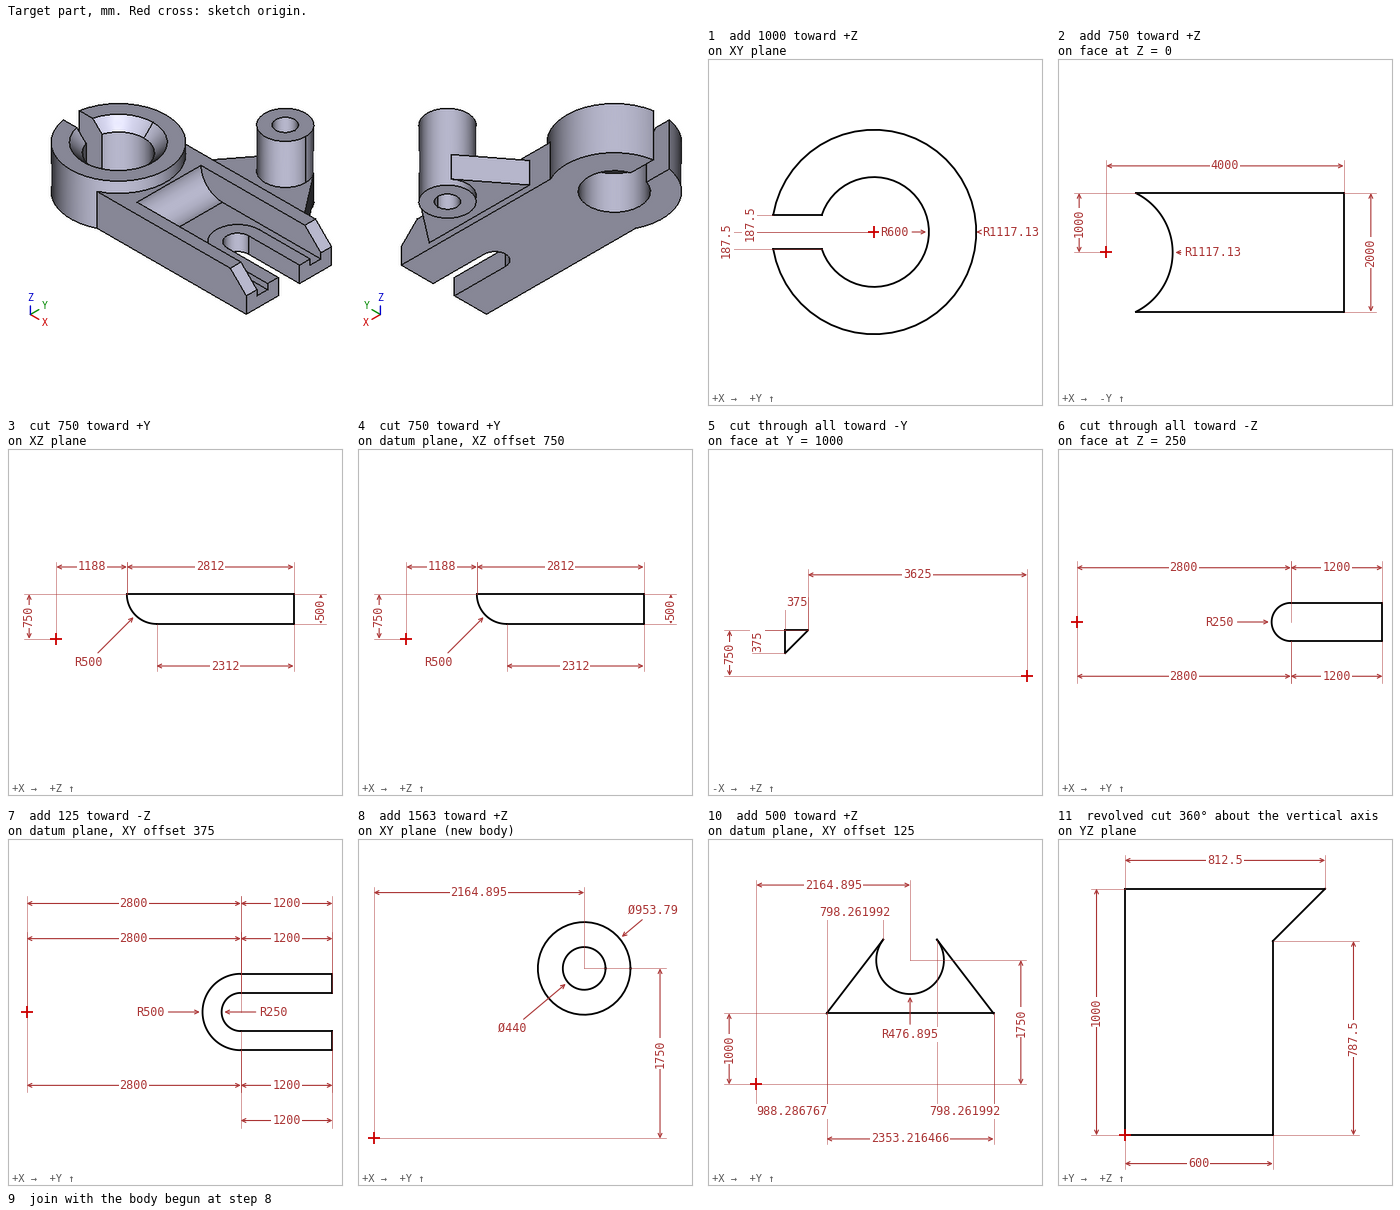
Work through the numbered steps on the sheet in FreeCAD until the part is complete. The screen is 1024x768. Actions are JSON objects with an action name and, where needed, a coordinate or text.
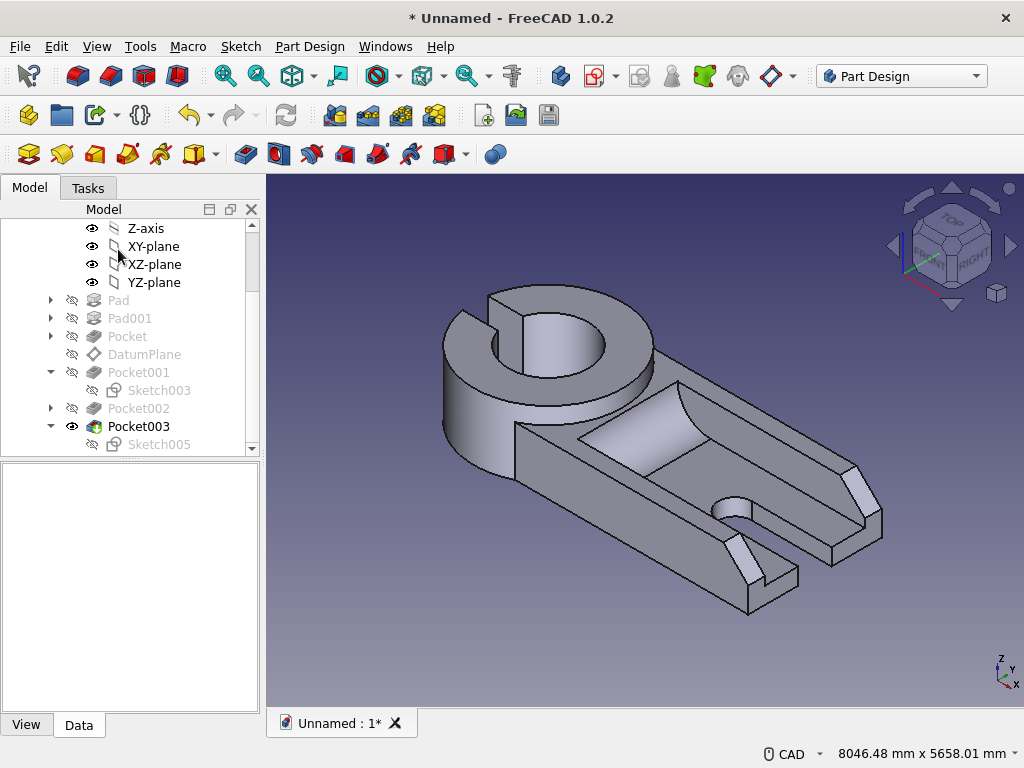
{"action": "scroll", "coordinate": [161, 332], "scroll_direction": "down", "scroll_amount": 3}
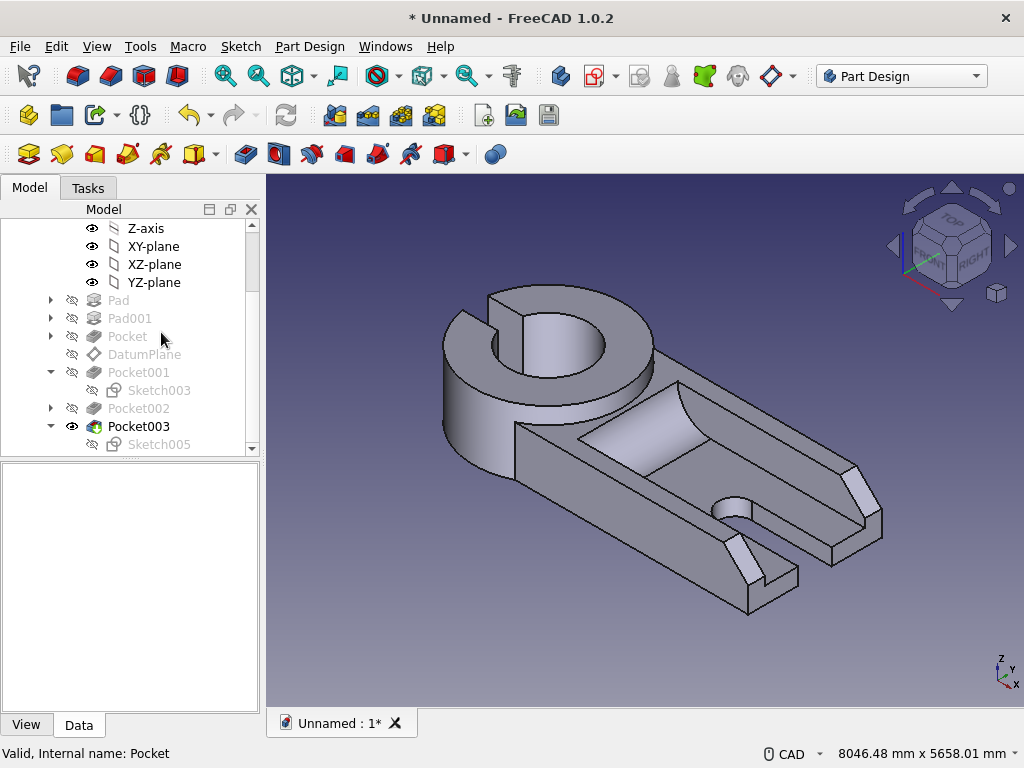
{"action": "scroll", "coordinate": [161, 332], "scroll_direction": "up", "scroll_amount": 15}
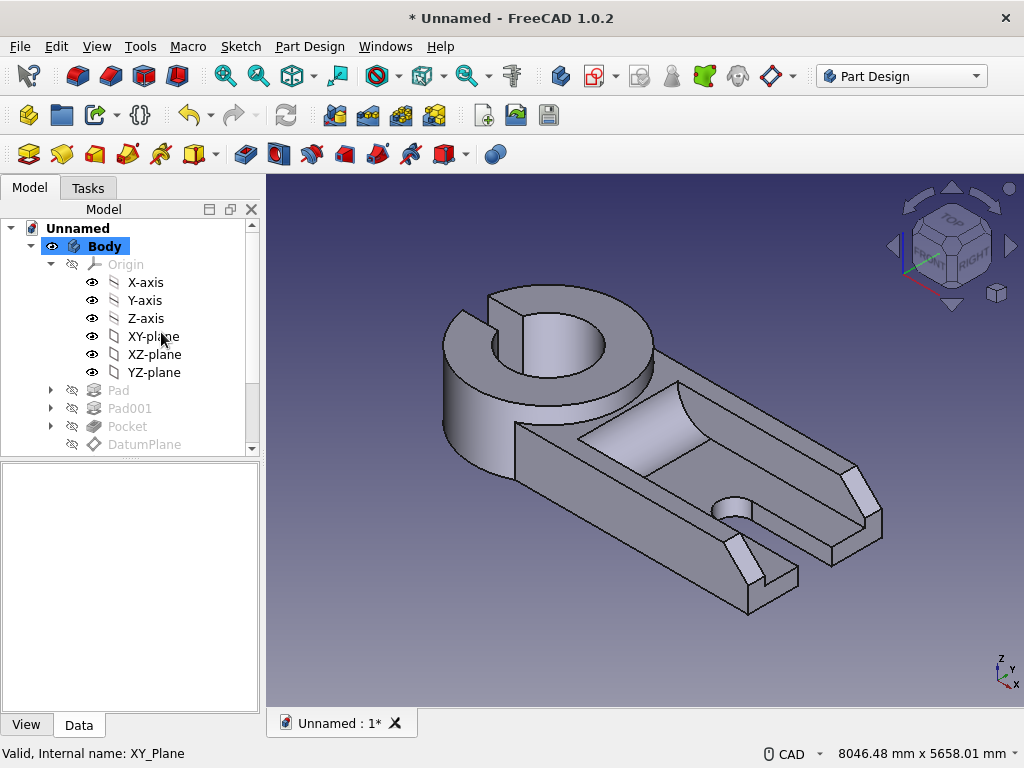
{"action": "left_click", "coordinate": [137, 336]}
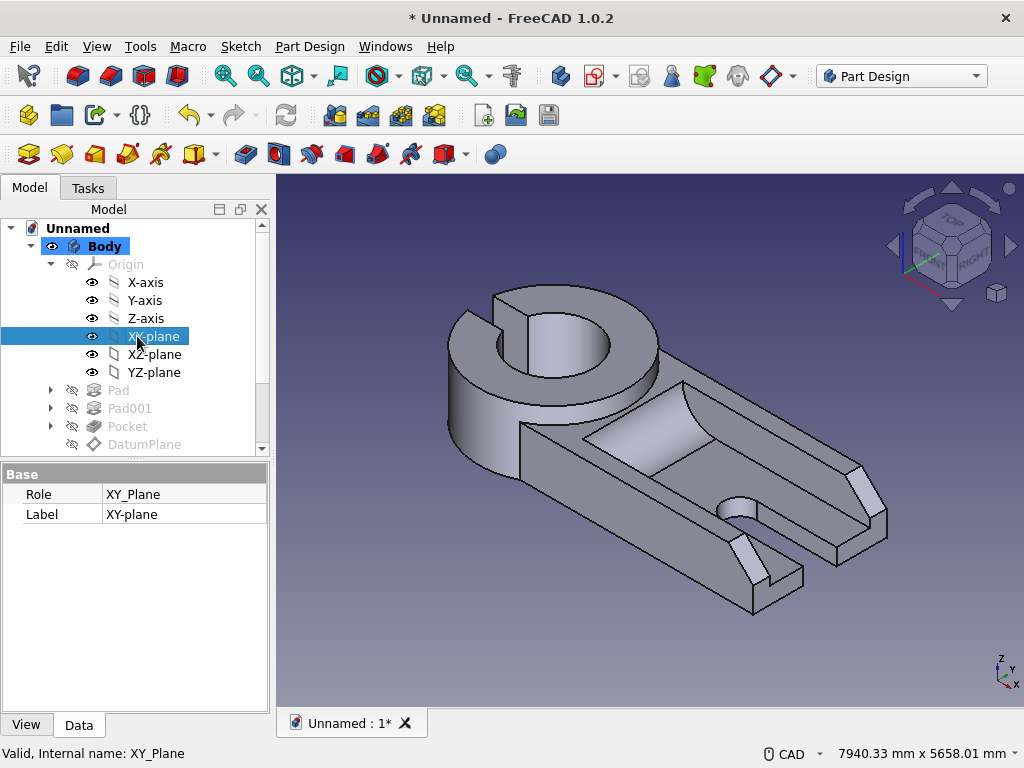
{"action": "left_click", "coordinate": [770, 76]}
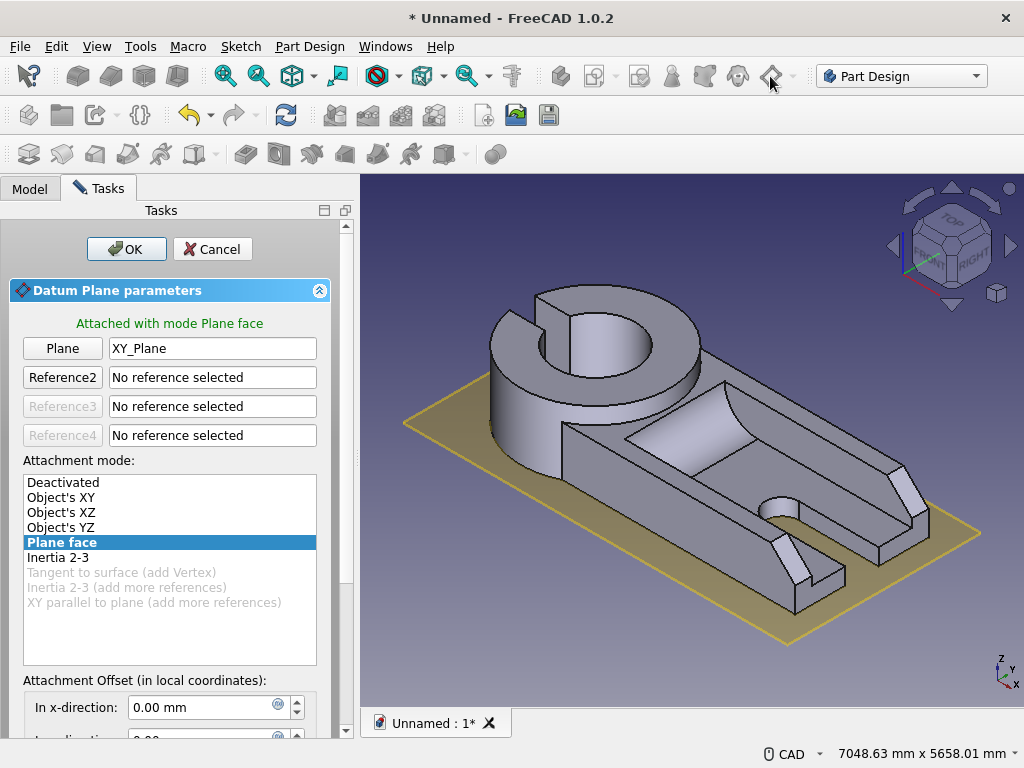
{"action": "scroll", "coordinate": [346, 479], "scroll_direction": "down", "scroll_amount": 2}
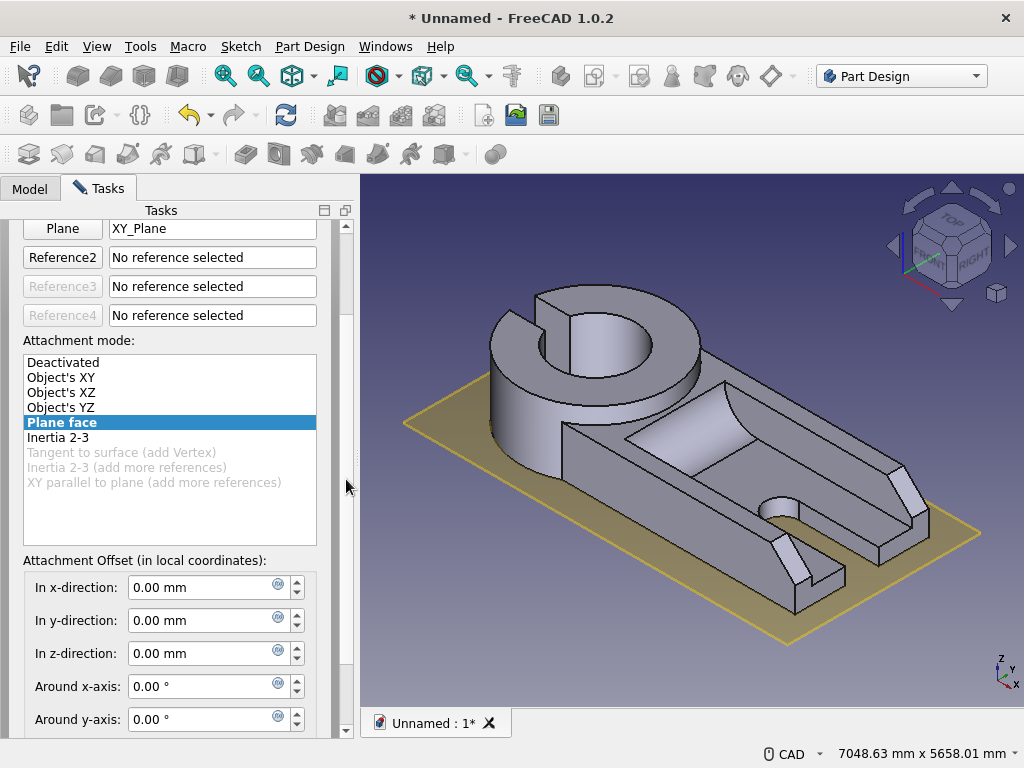
{"action": "triple_click", "coordinate": [210, 654]}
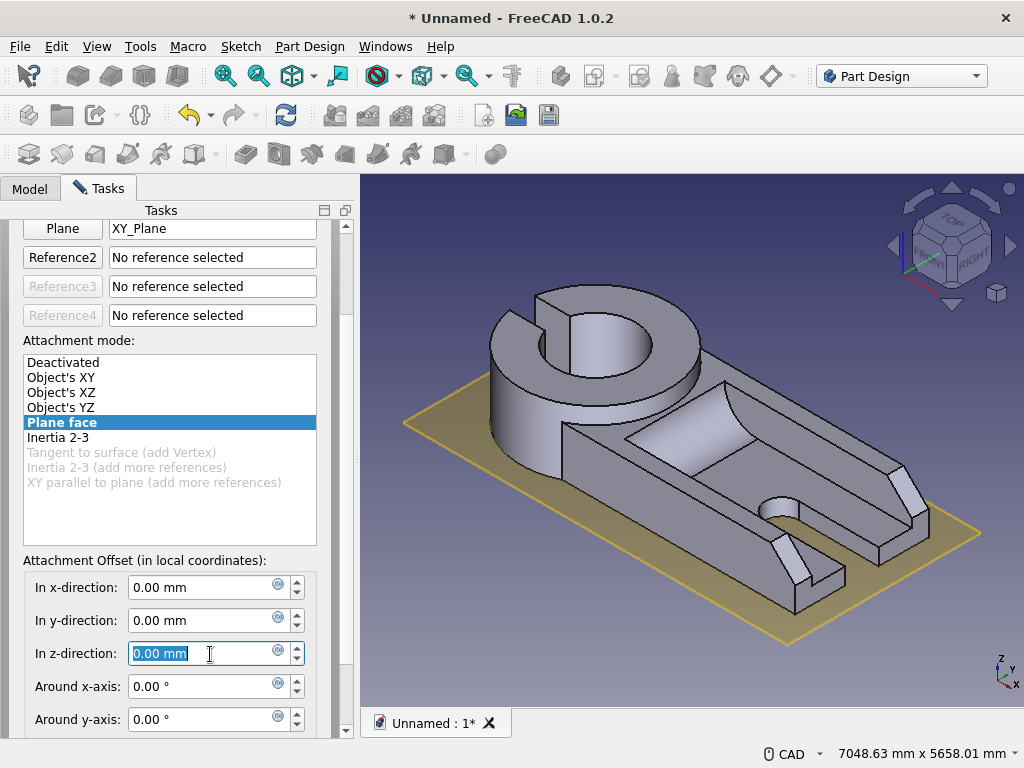
{"action": "type", "text": "375"}
{"action": "key", "text": "Tab"}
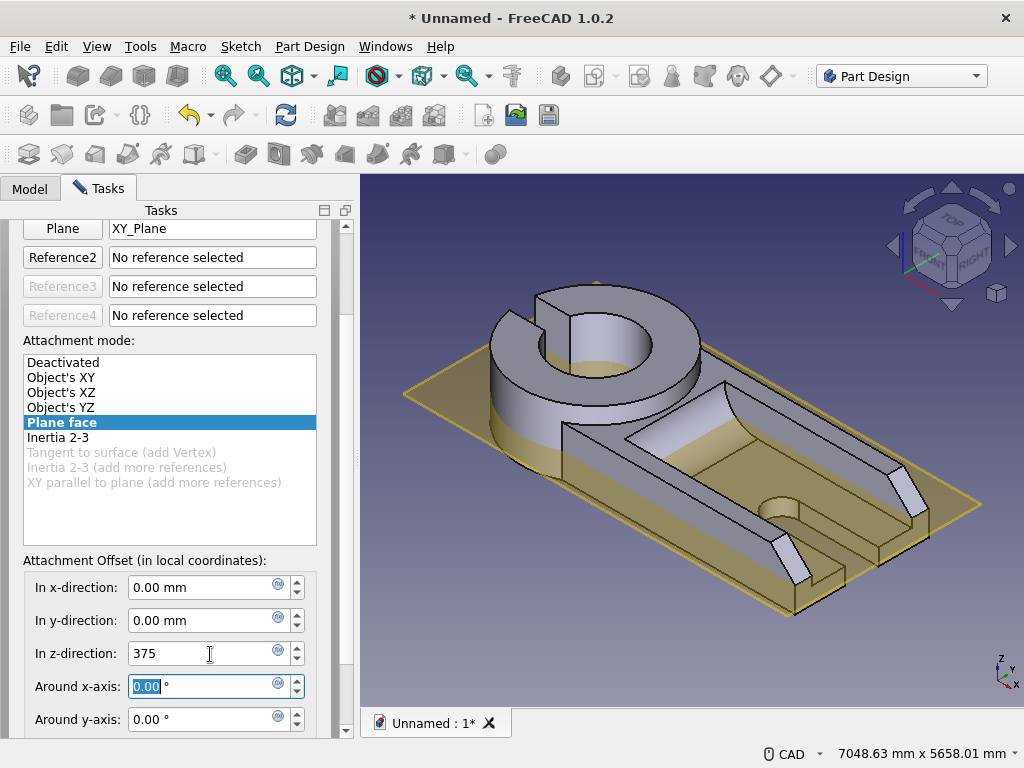
{"action": "scroll", "coordinate": [346, 479], "scroll_direction": "up", "scroll_amount": 3}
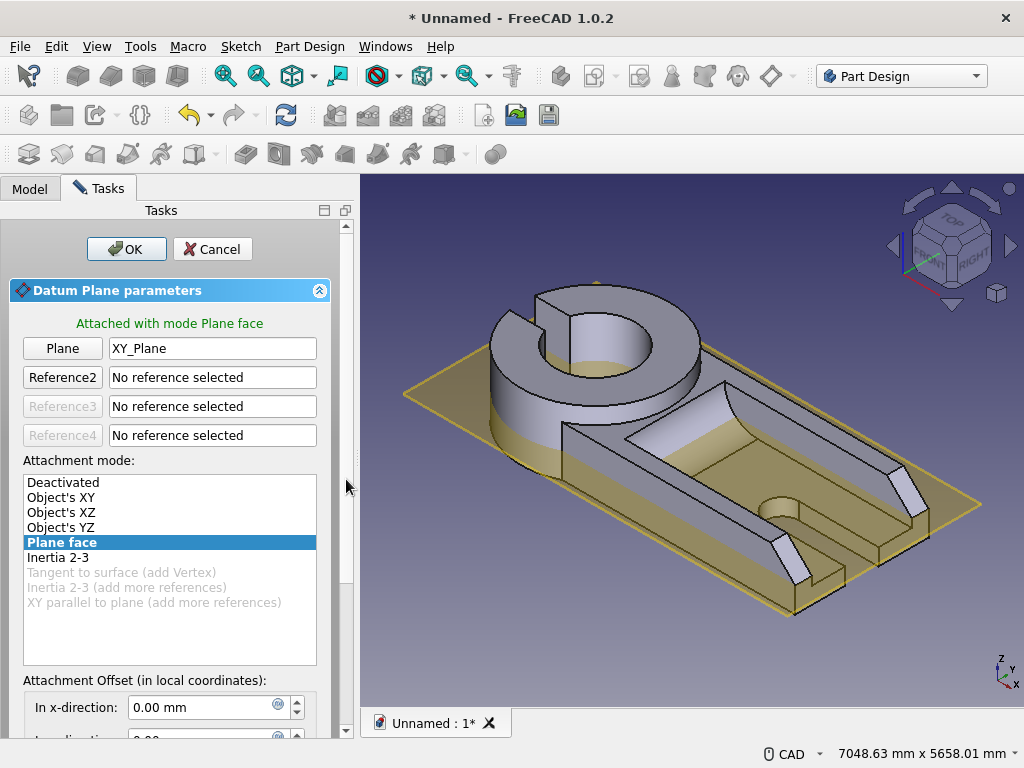
{"action": "left_click", "coordinate": [127, 249]}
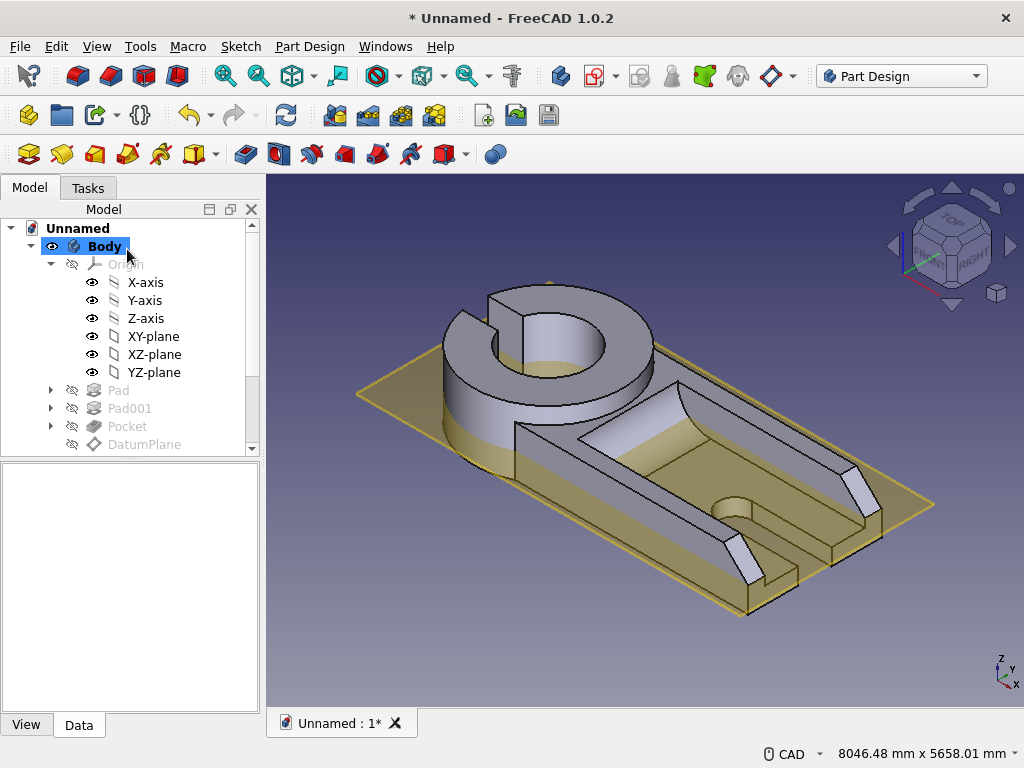
{"action": "scroll", "coordinate": [101, 332], "scroll_direction": "down", "scroll_amount": 3}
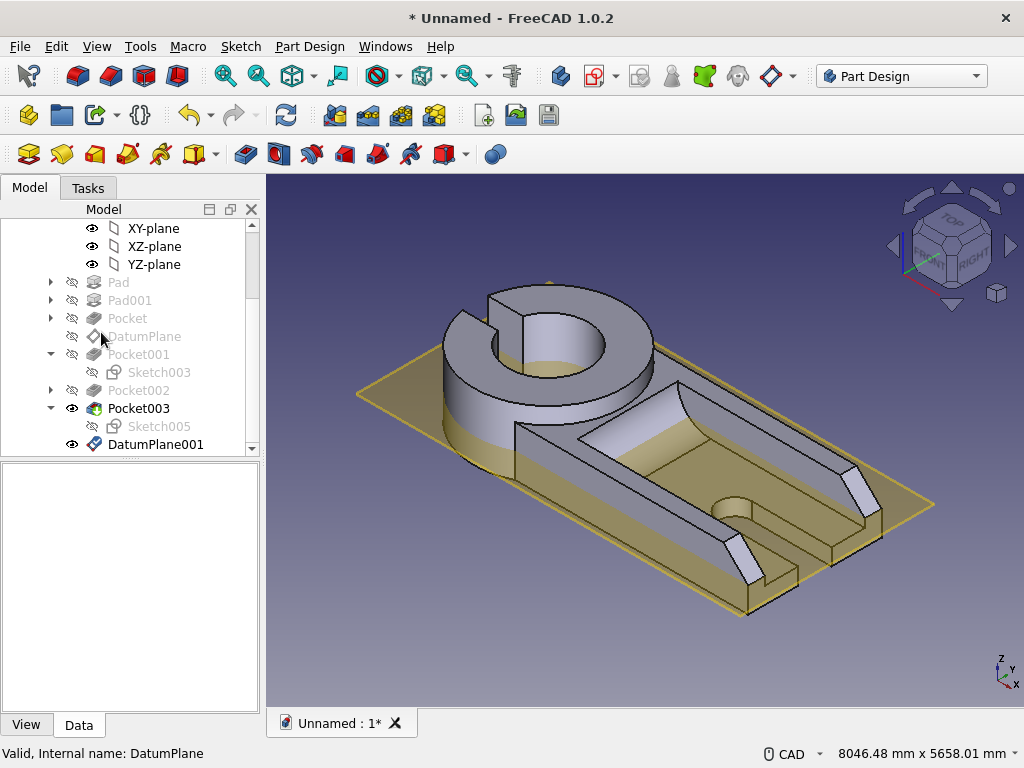
{"action": "left_click", "coordinate": [117, 444]}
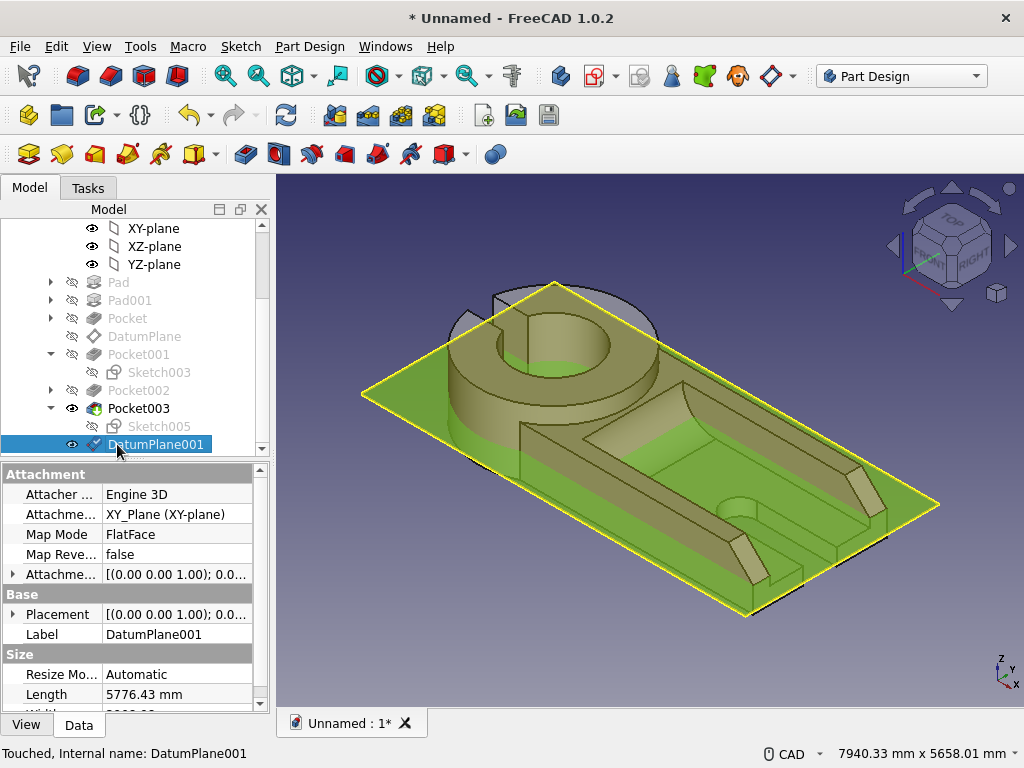
{"action": "left_click", "coordinate": [594, 76]}